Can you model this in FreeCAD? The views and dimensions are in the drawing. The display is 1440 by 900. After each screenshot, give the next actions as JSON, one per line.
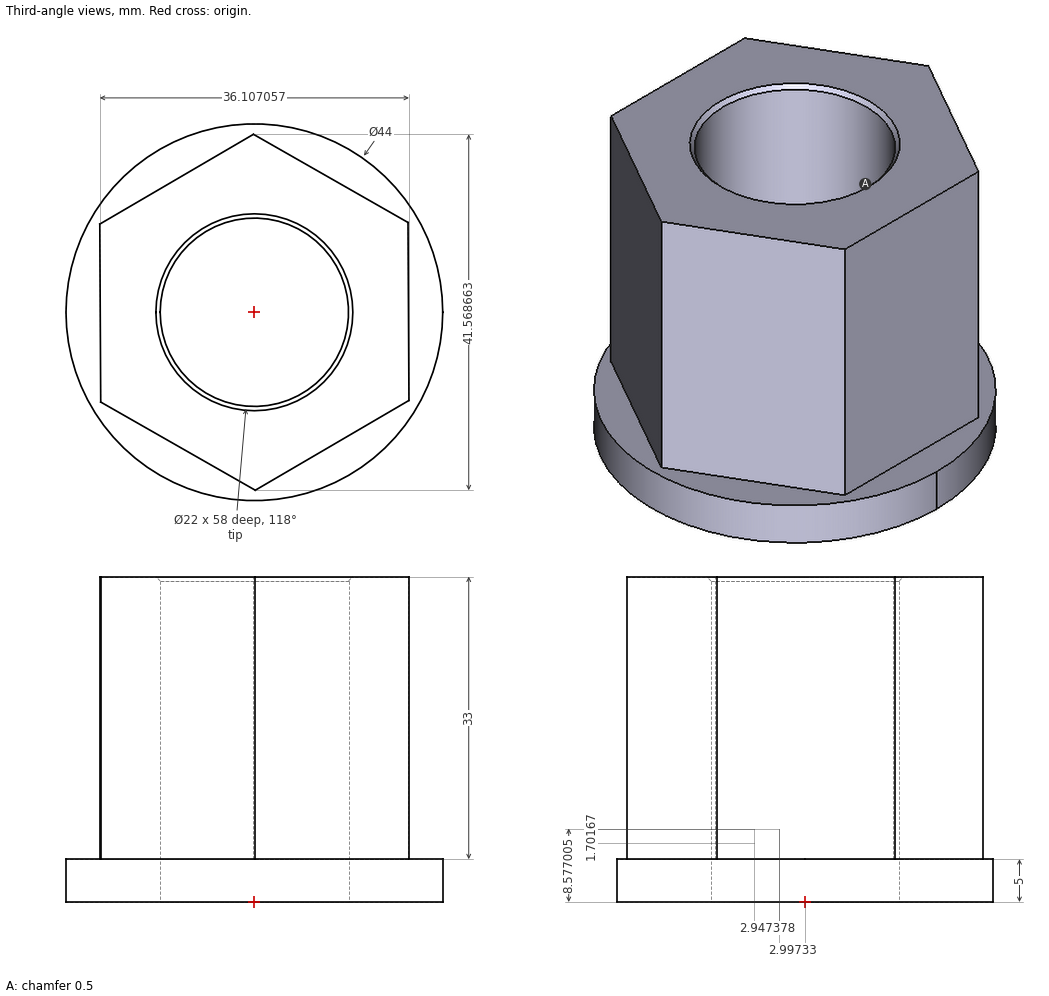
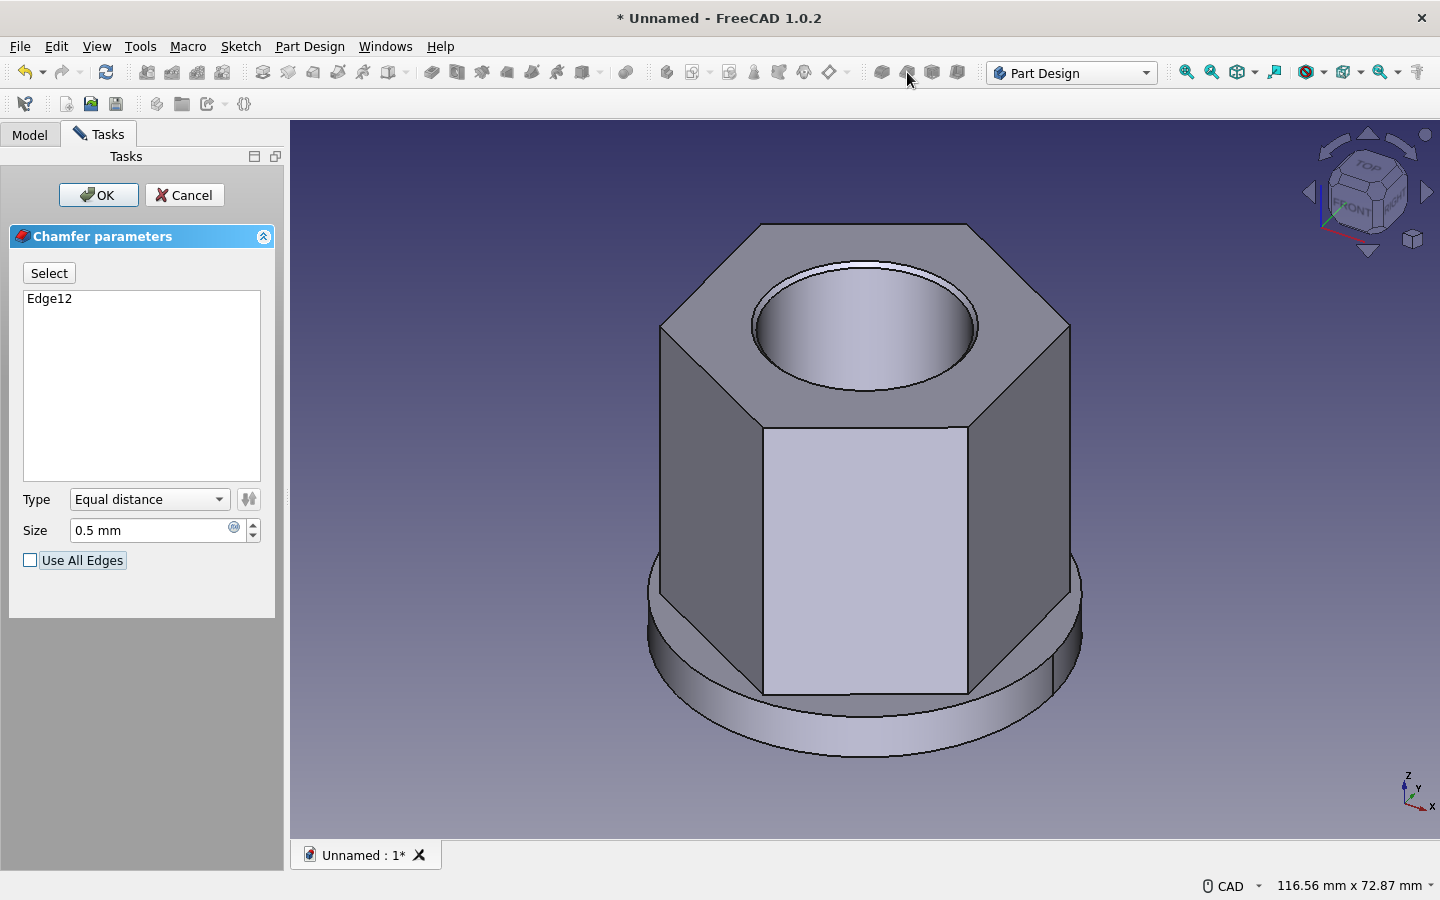
{"action": "left_click", "coordinate": [99, 195]}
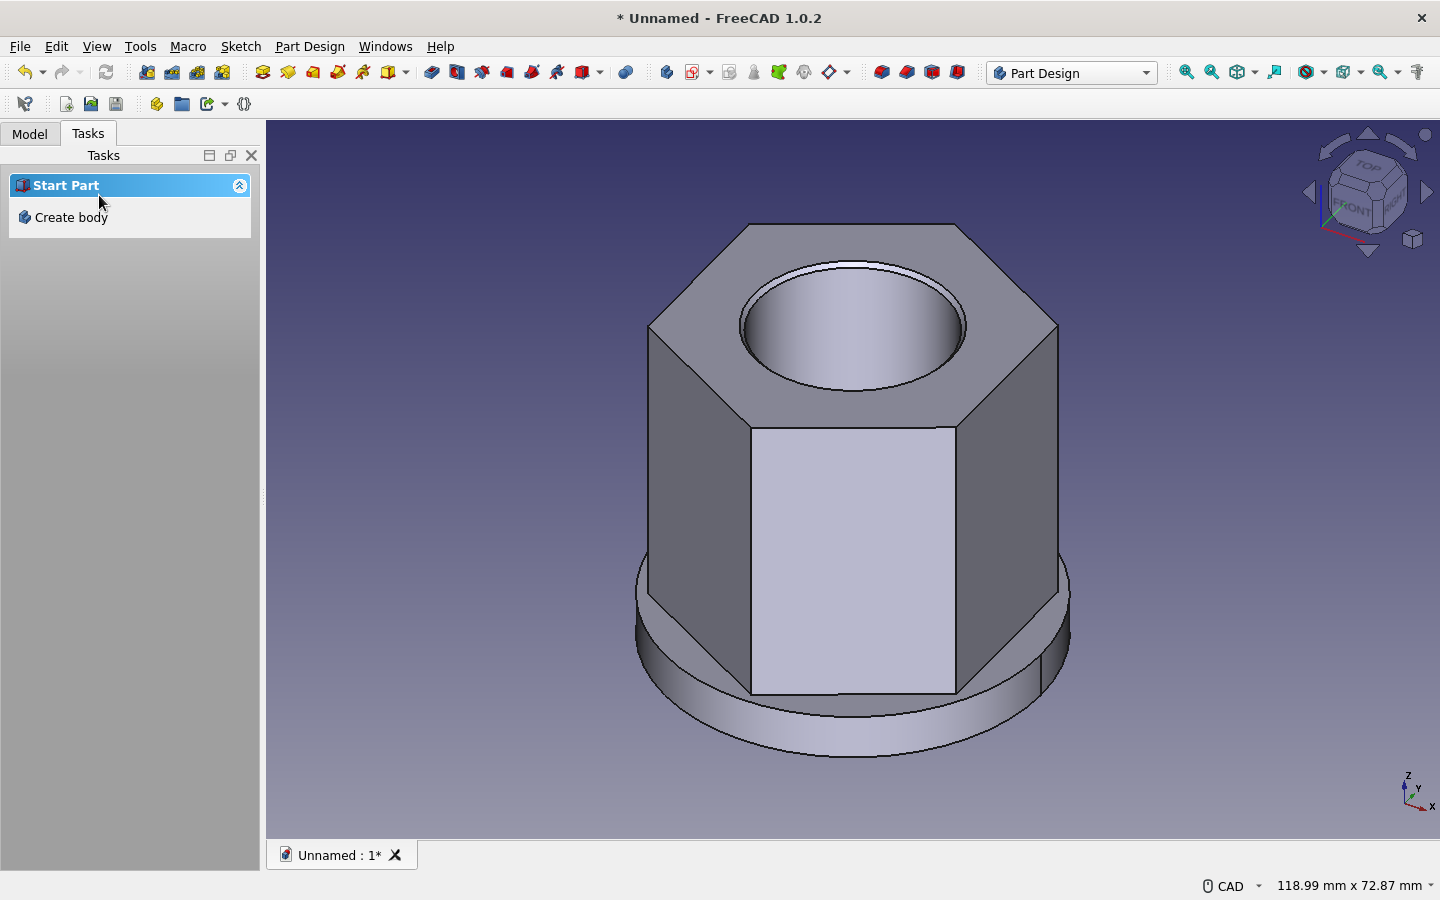
{"action": "key", "text": "0"}